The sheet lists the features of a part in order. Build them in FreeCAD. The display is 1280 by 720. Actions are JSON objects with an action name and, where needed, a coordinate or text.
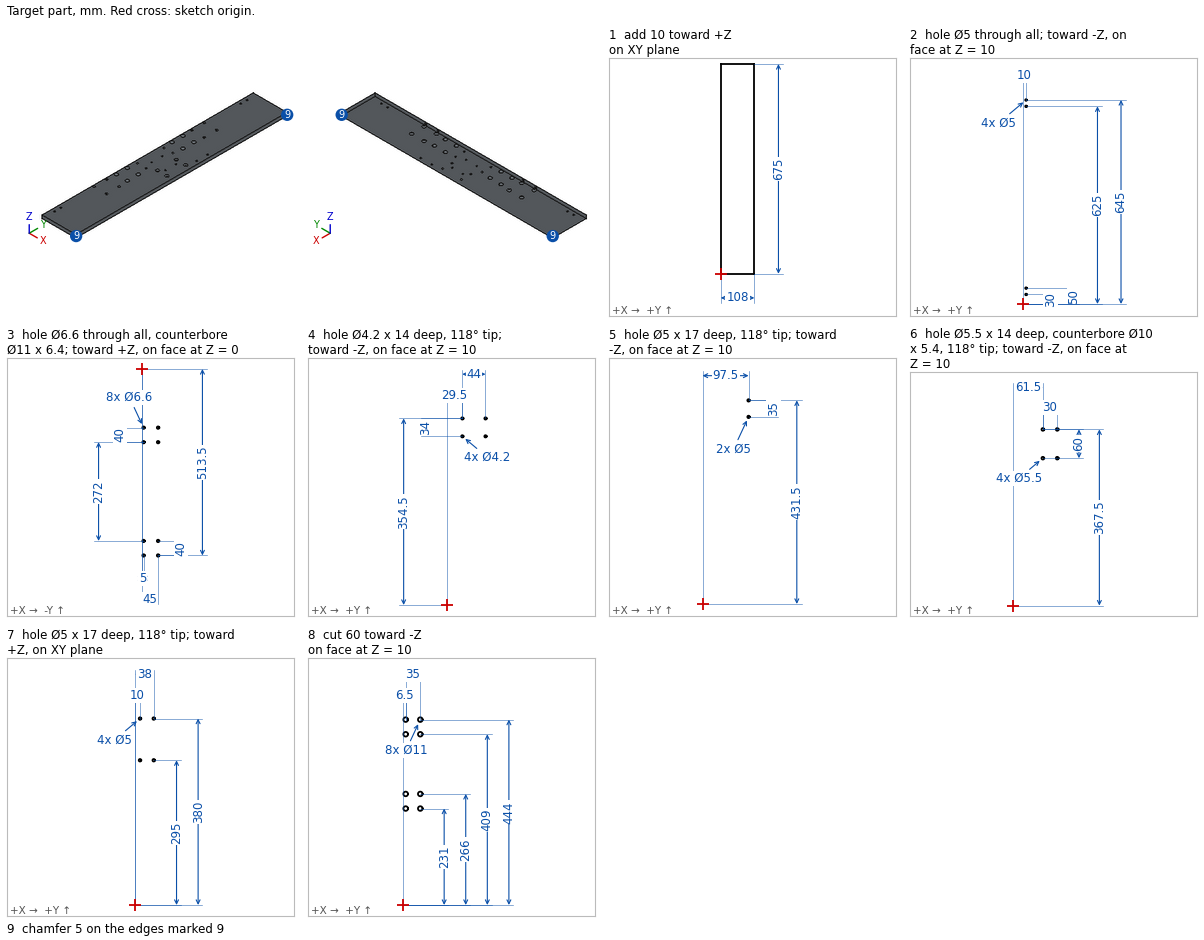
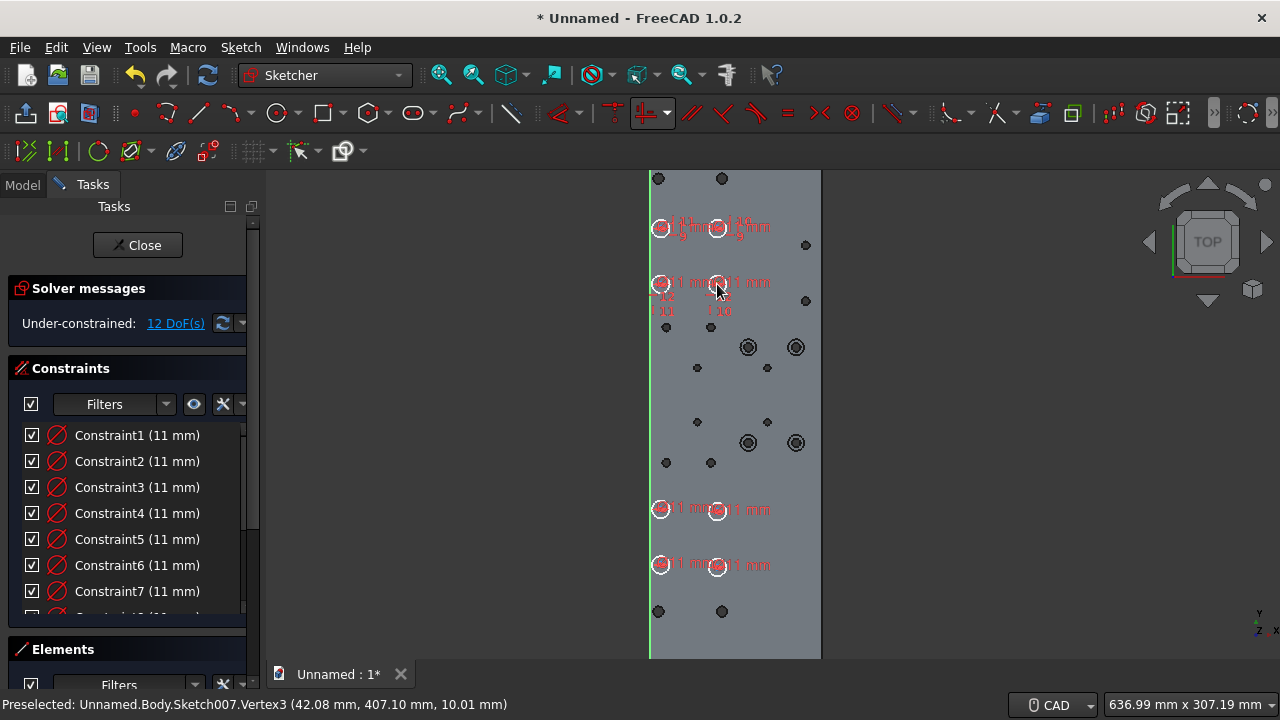
{"action": "left_click", "coordinate": [717, 512]}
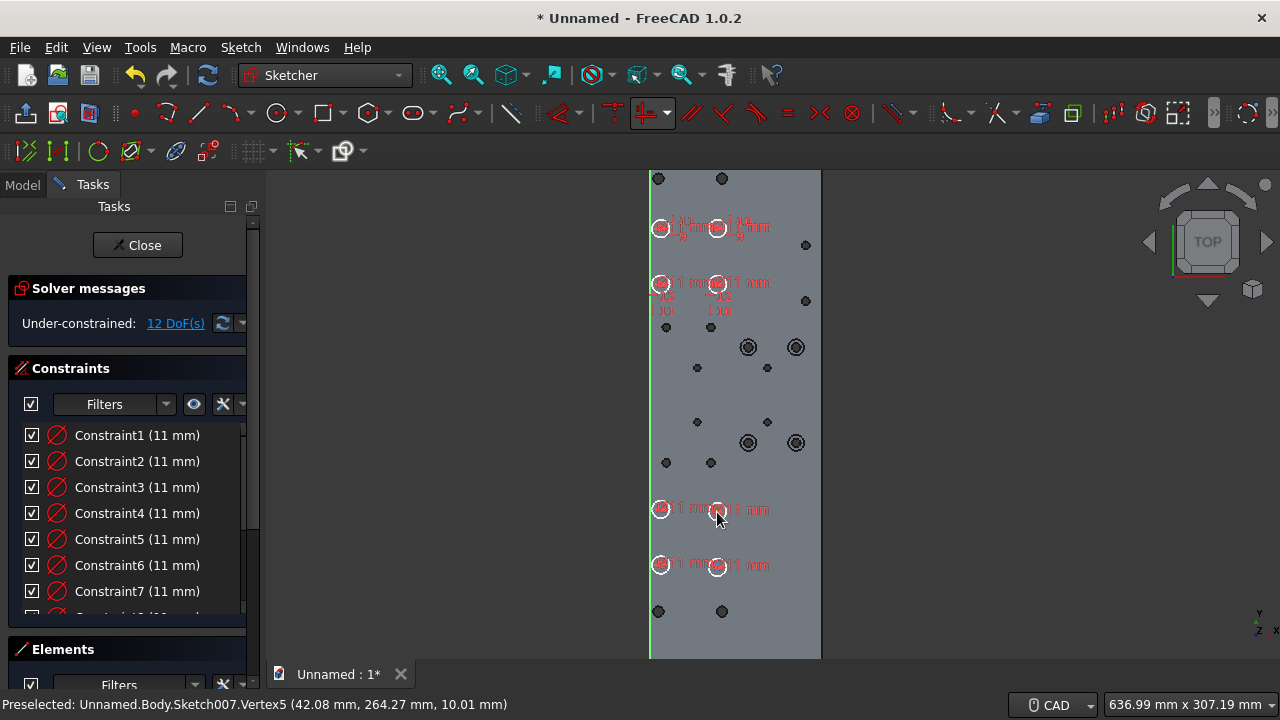
{"action": "key", "text": "v"}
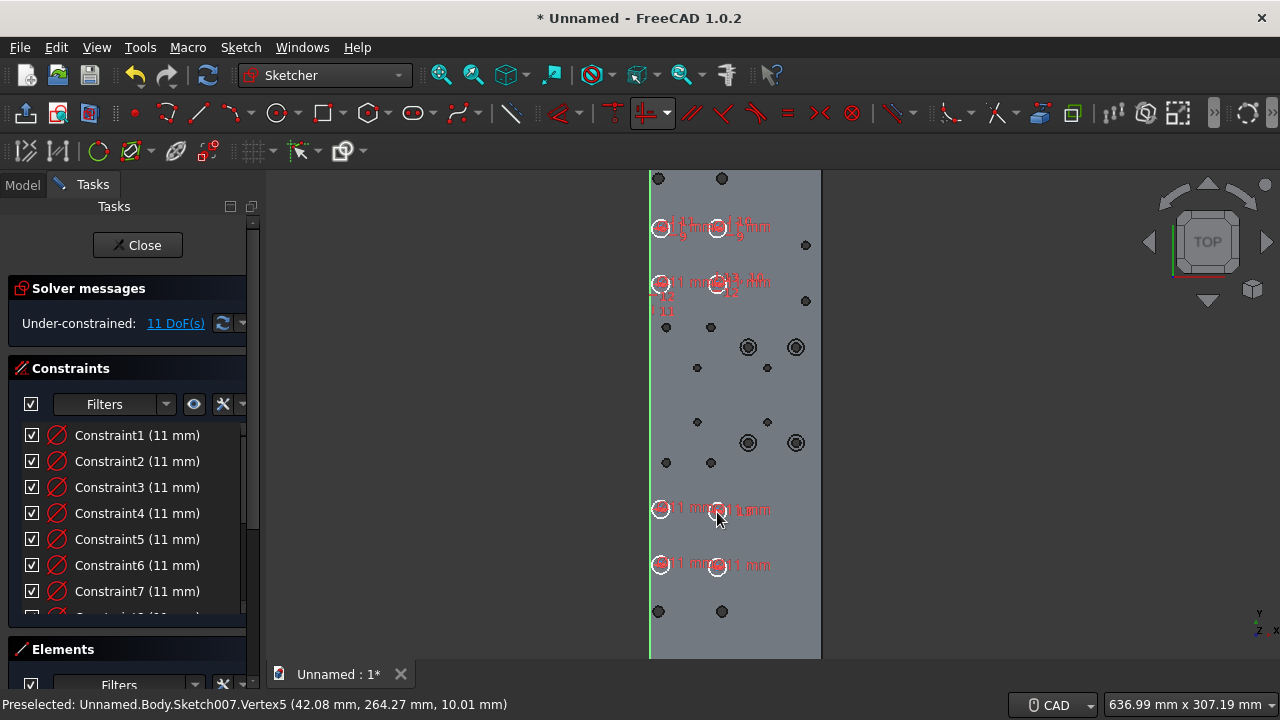
{"action": "left_click", "coordinate": [717, 512]}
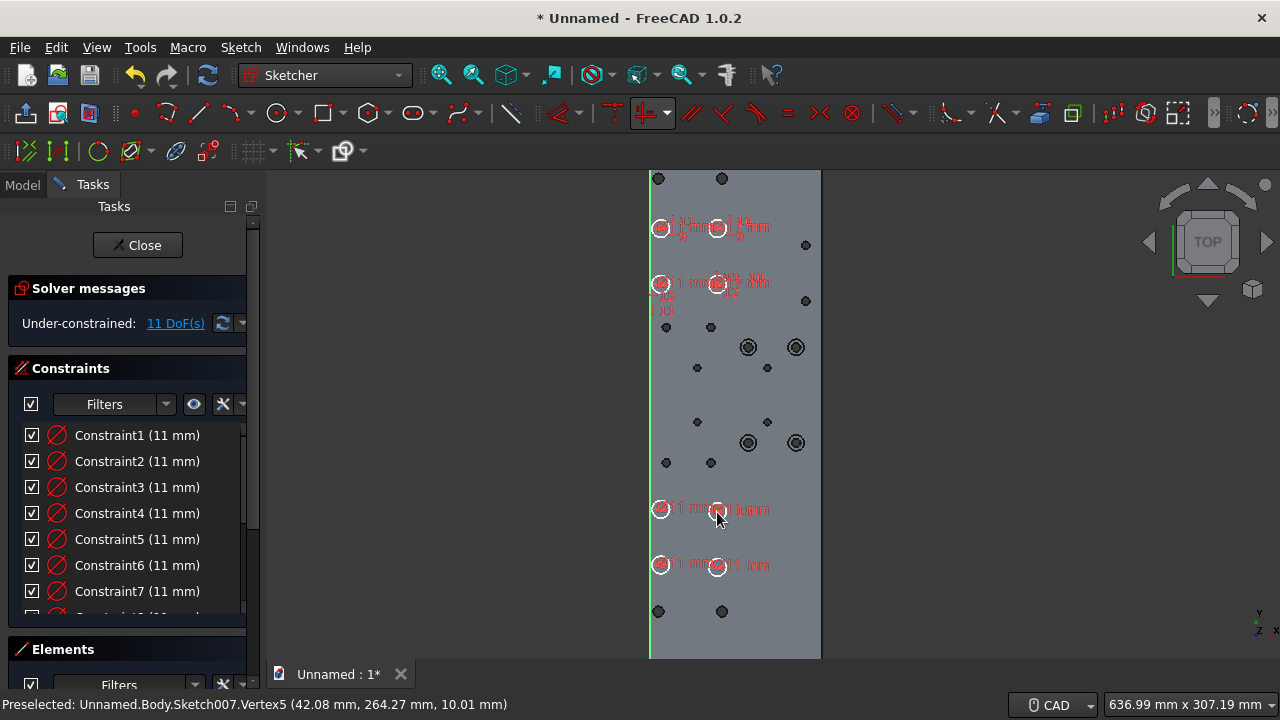
{"action": "left_click", "coordinate": [717, 567]}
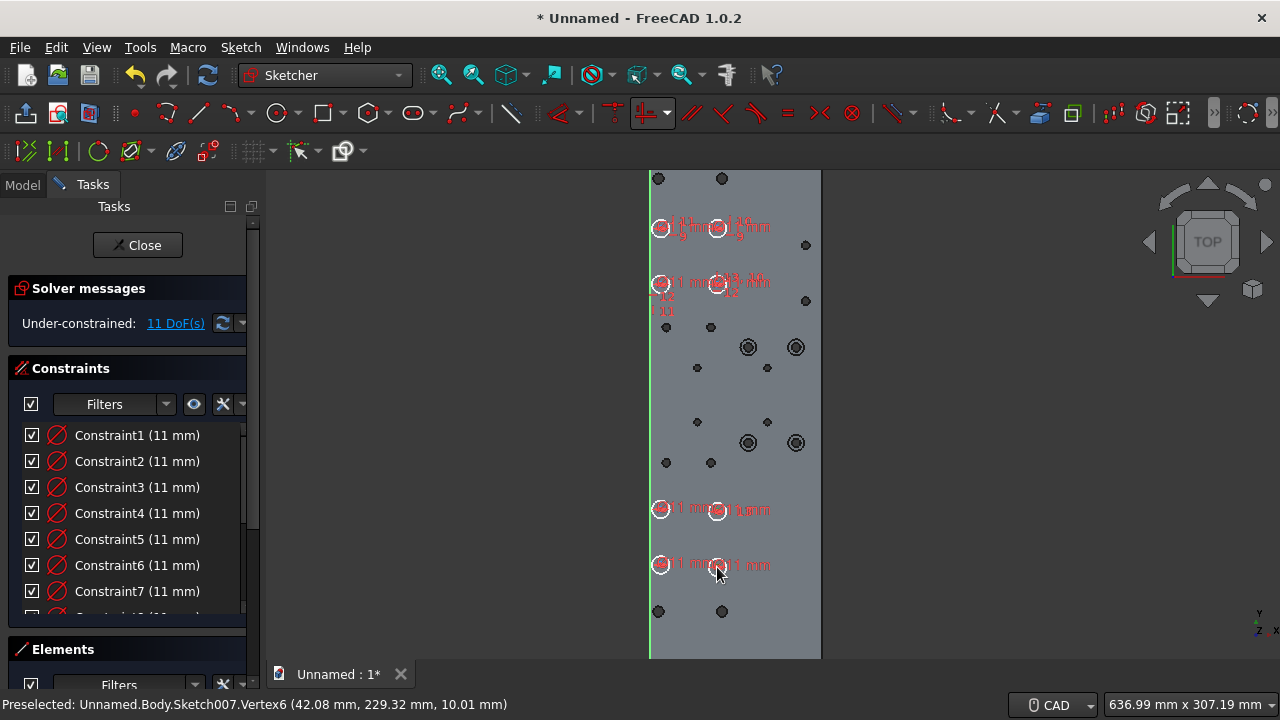
{"action": "left_click", "coordinate": [670, 114]}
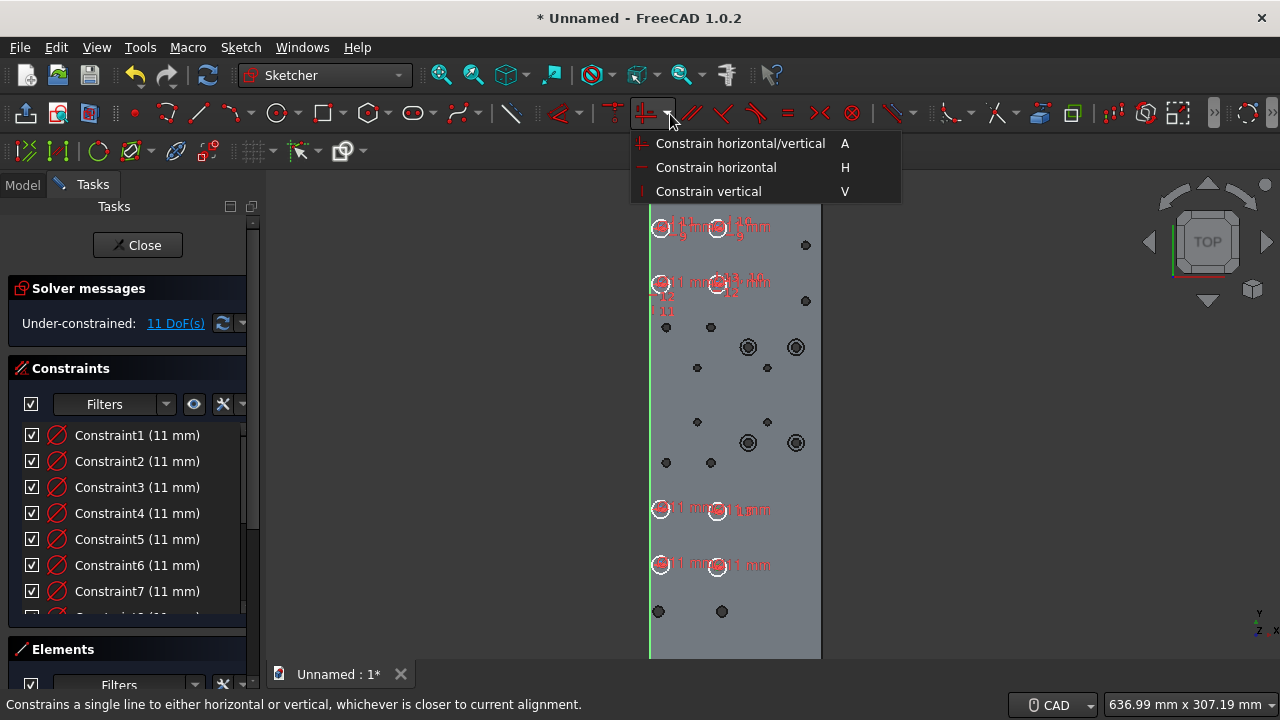
{"action": "left_click", "coordinate": [766, 191]}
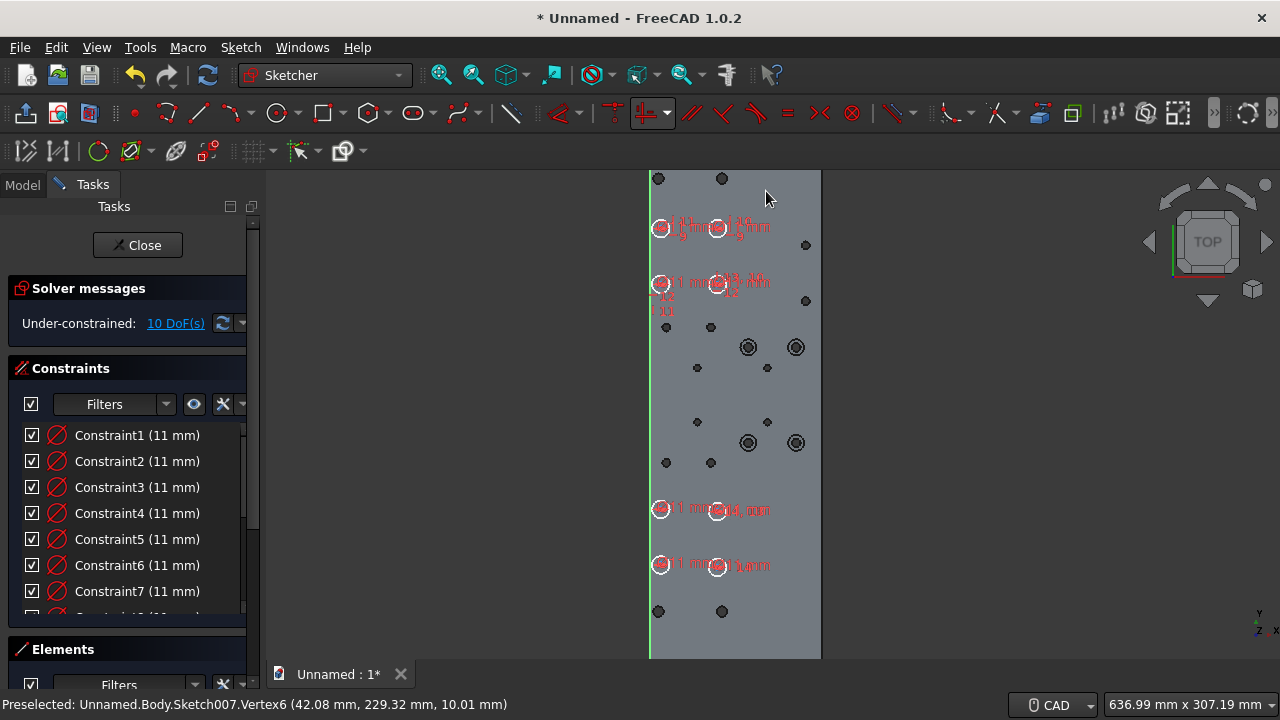
{"action": "left_click", "coordinate": [661, 284]}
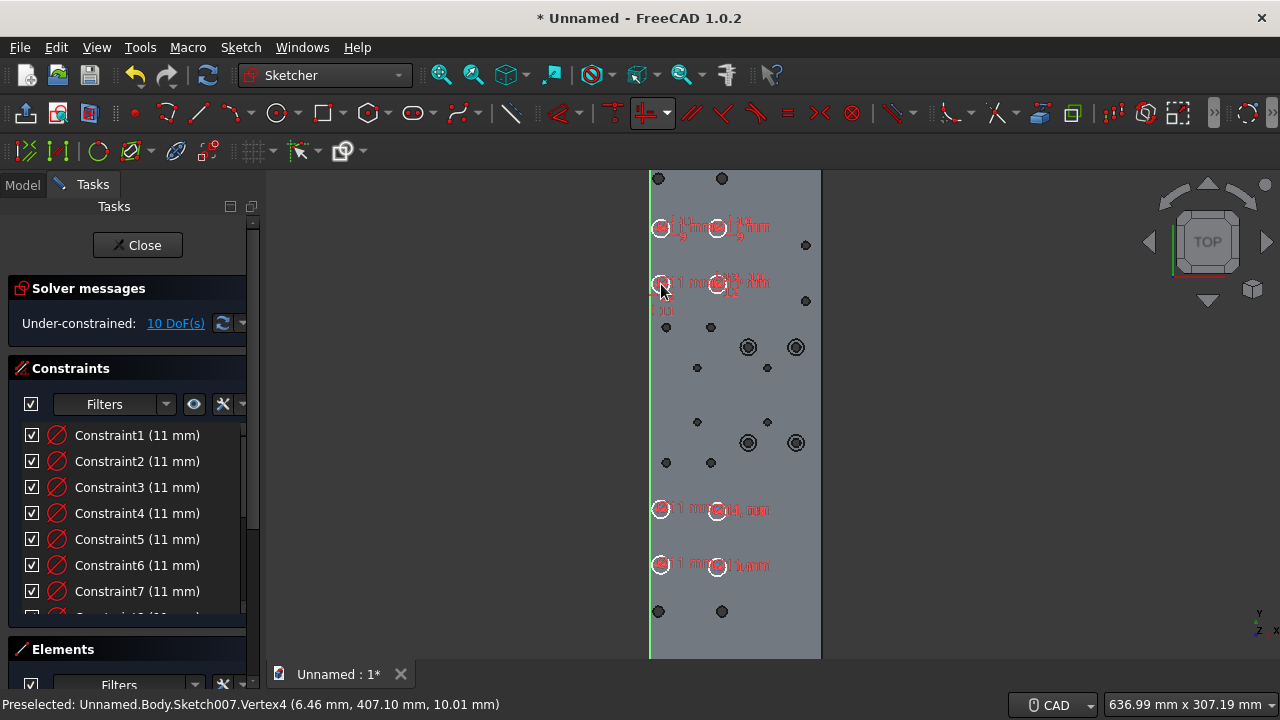
{"action": "left_click", "coordinate": [661, 565]}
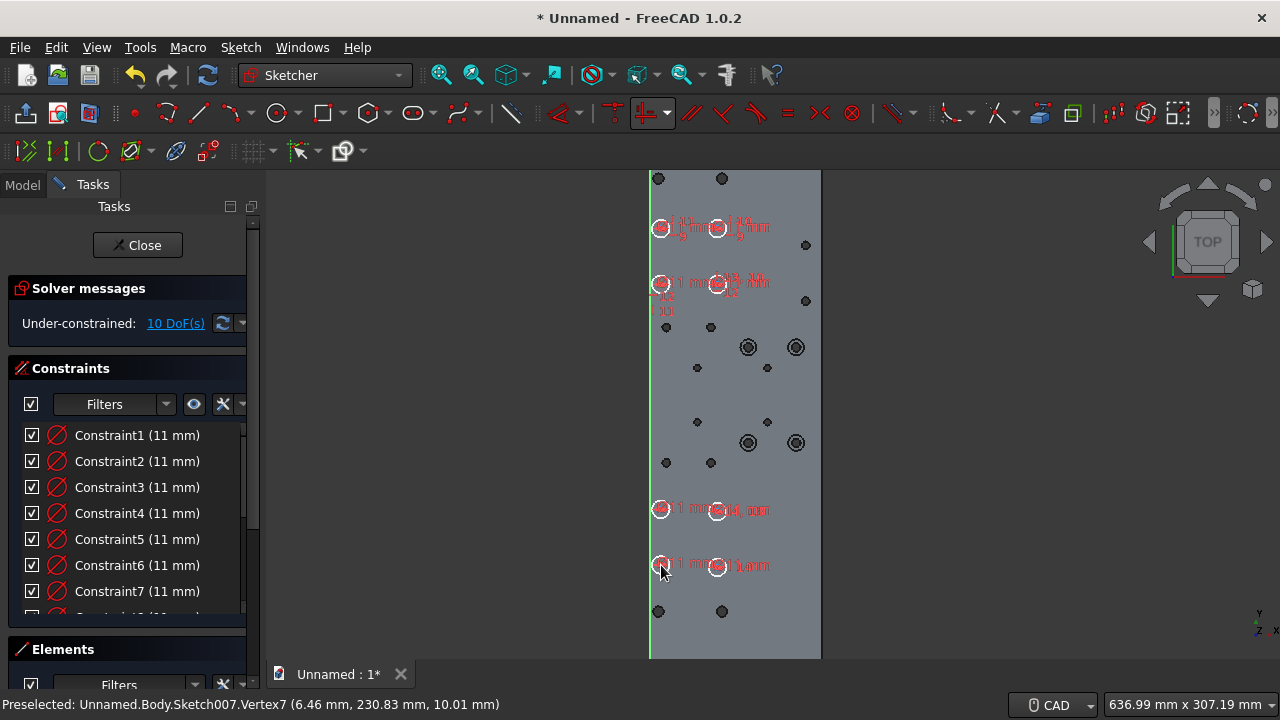
{"action": "left_click", "coordinate": [670, 114]}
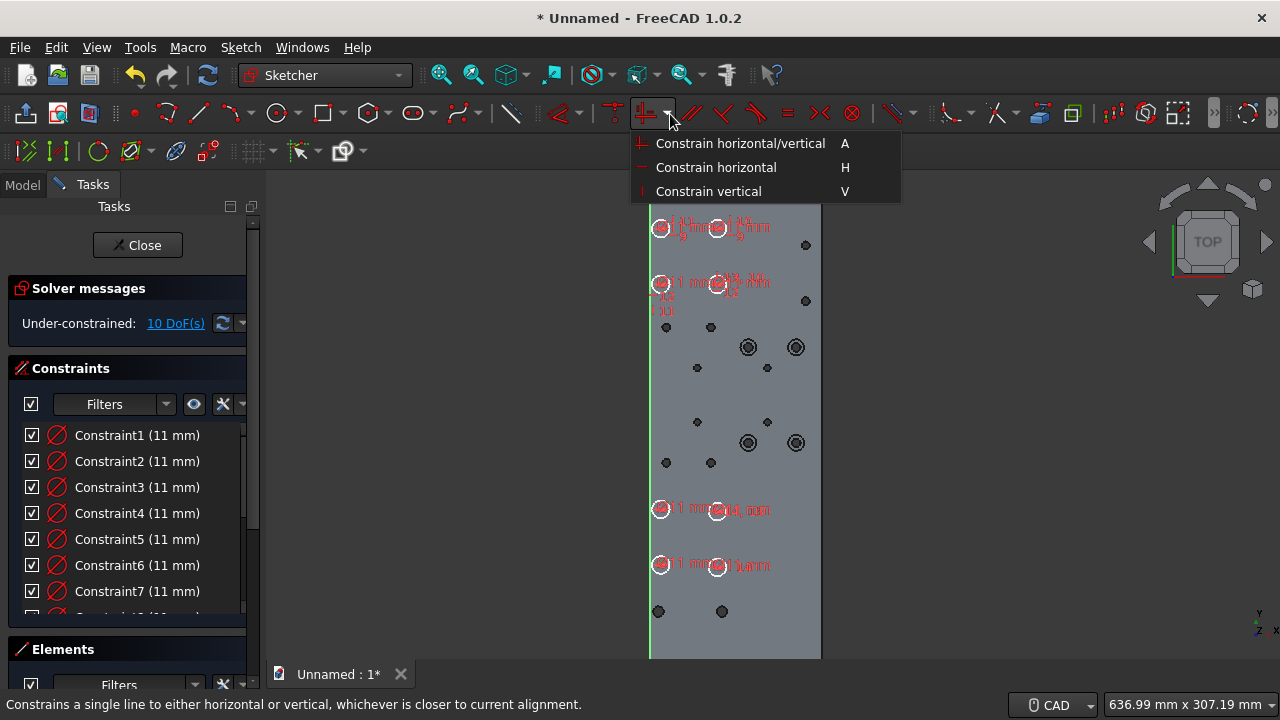
{"action": "left_click", "coordinate": [766, 191]}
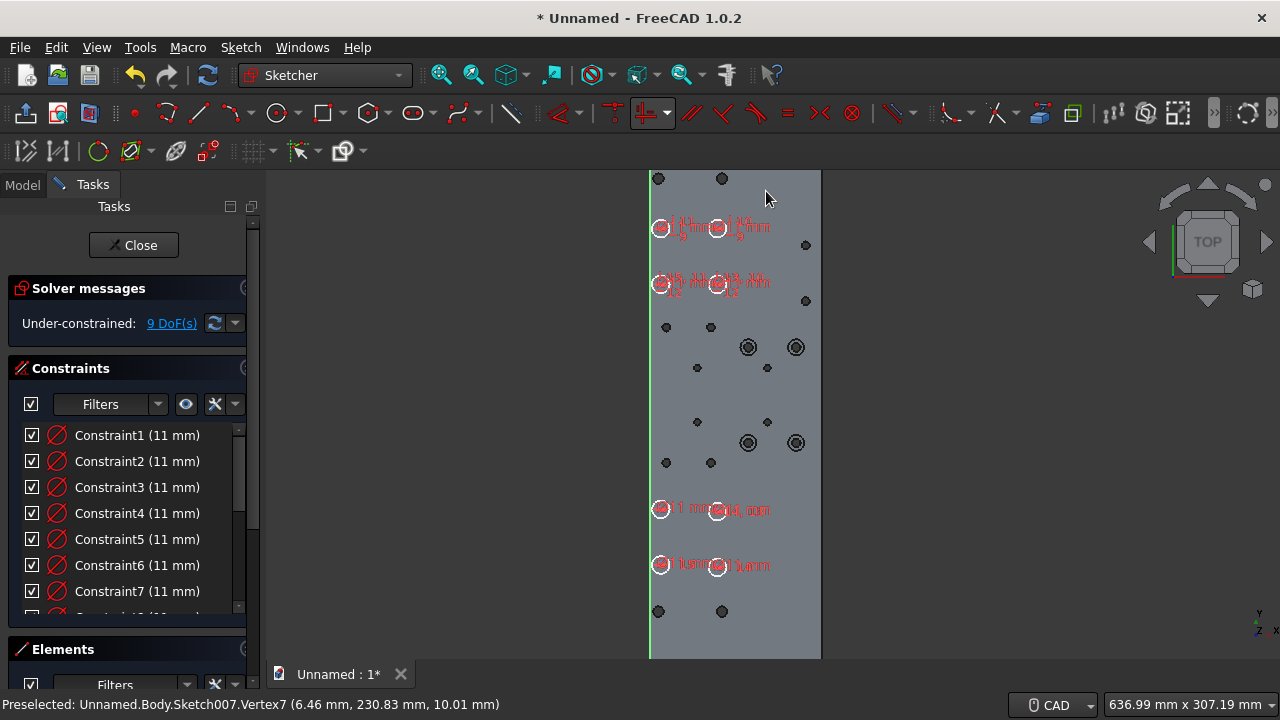
{"action": "left_click", "coordinate": [717, 567]}